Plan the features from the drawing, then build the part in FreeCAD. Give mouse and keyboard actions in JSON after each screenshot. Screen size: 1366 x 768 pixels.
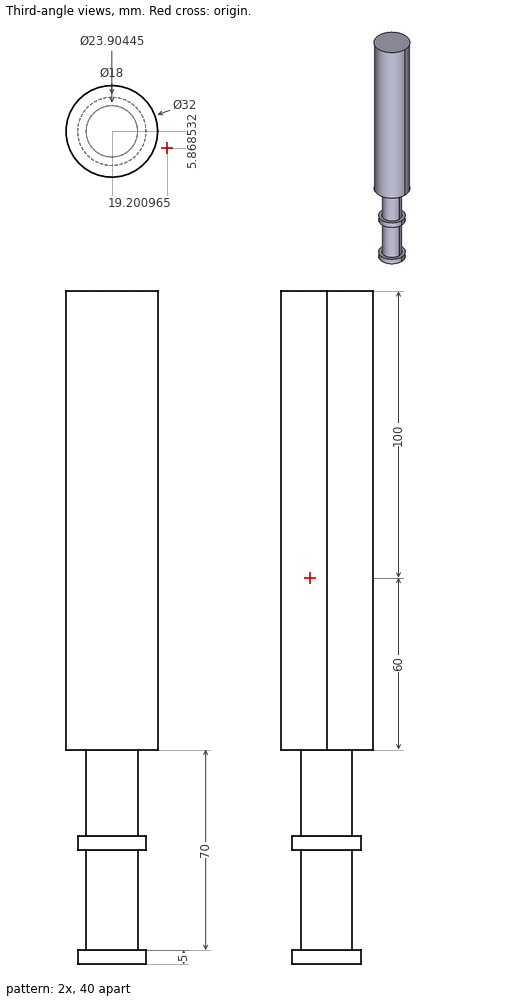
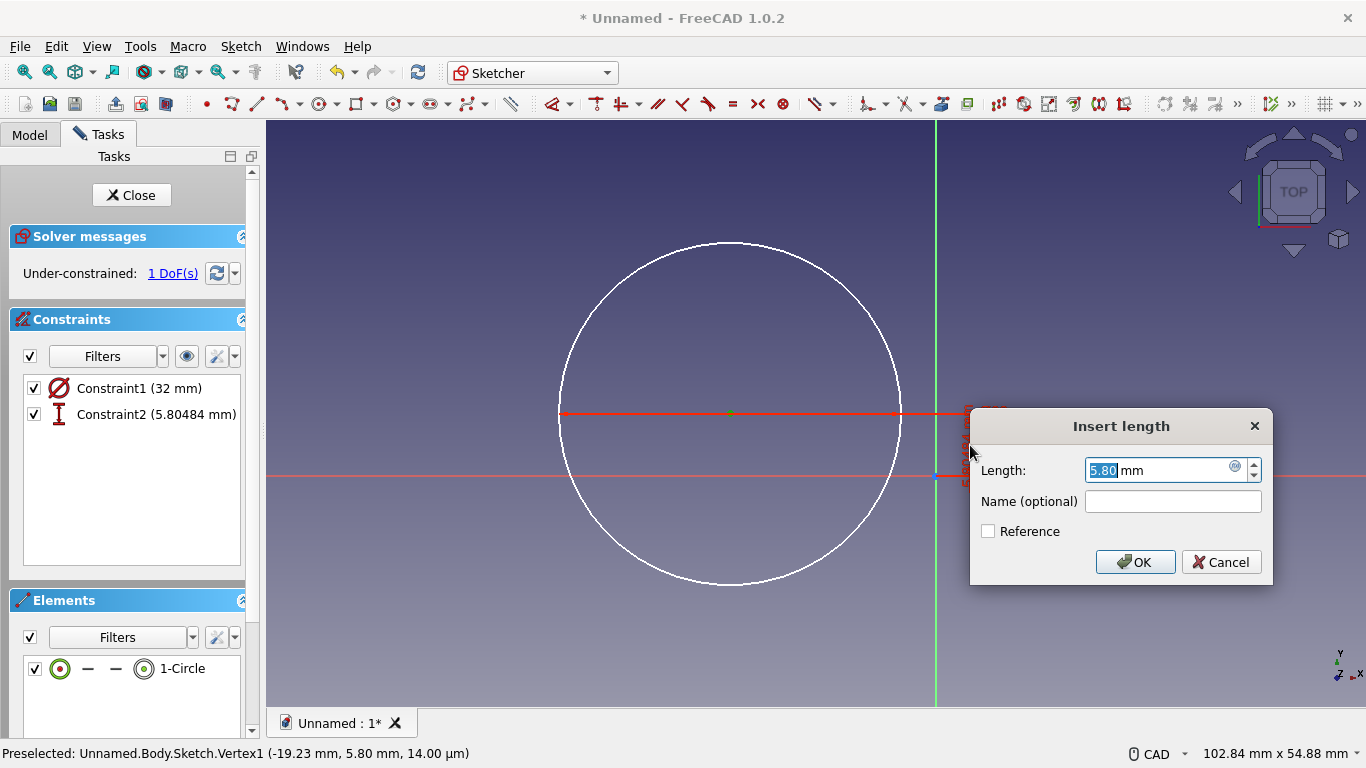
{"action": "type", "text": "5.868532"}
{"action": "key", "text": "Return"}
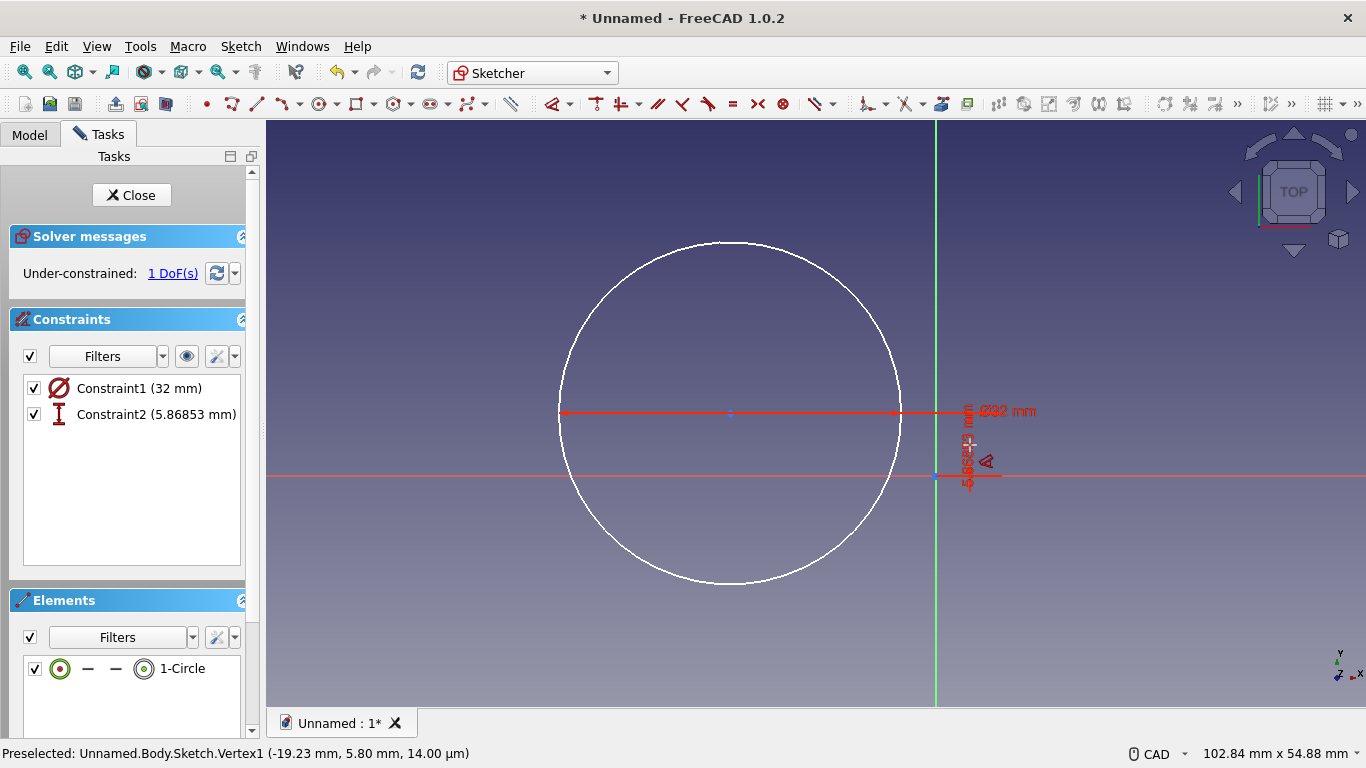
{"action": "left_click", "coordinate": [730, 413]}
{"action": "left_click", "coordinate": [833, 510]}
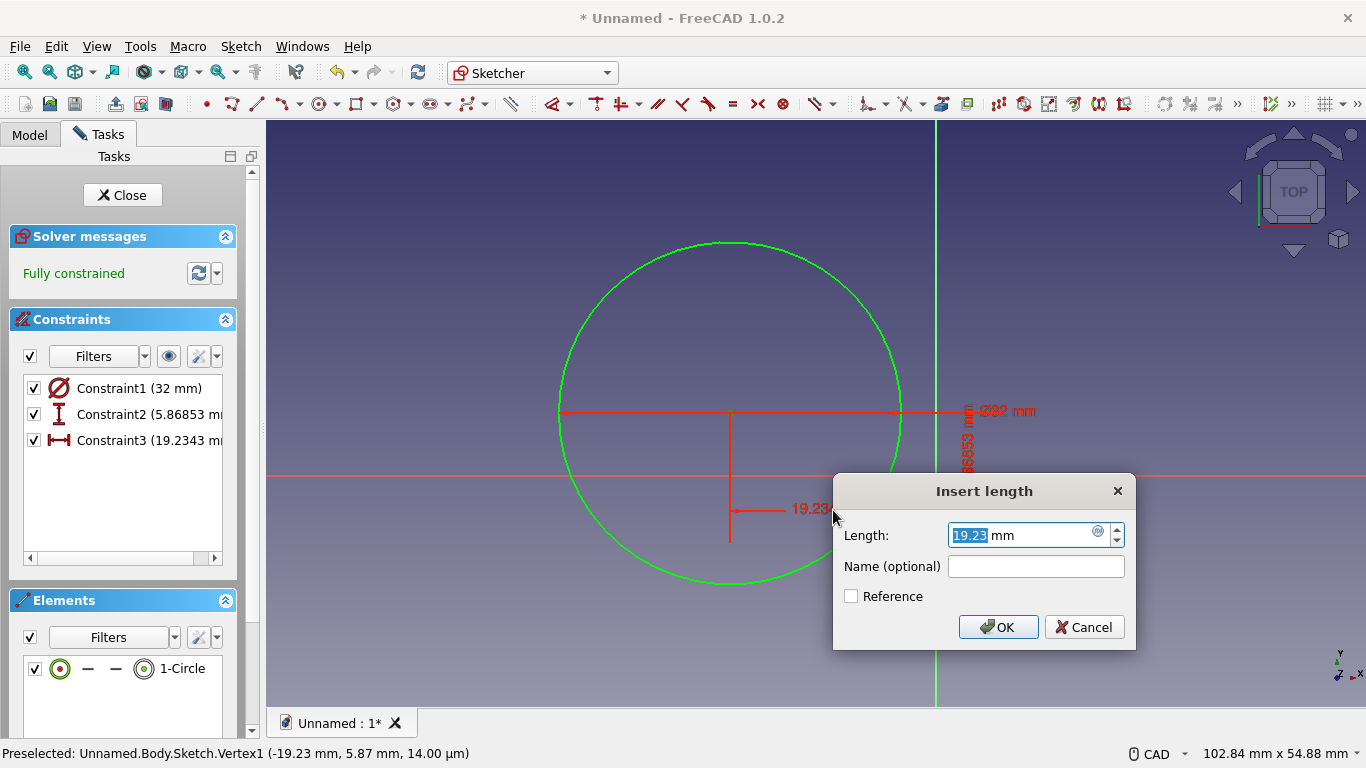
{"action": "type", "text": "19.200965"}
{"action": "key", "text": "Return"}
{"action": "key", "text": "Escape"}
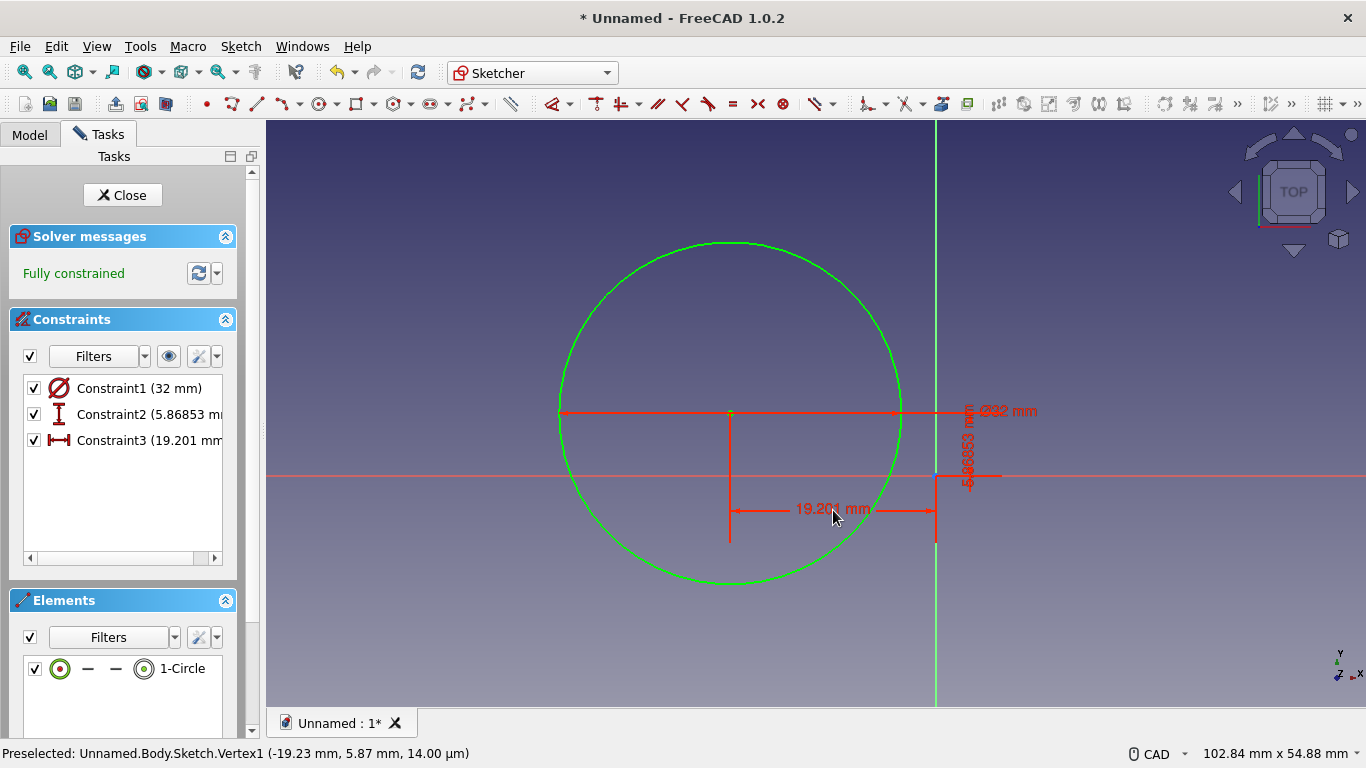
{"action": "left_click", "coordinate": [123, 195]}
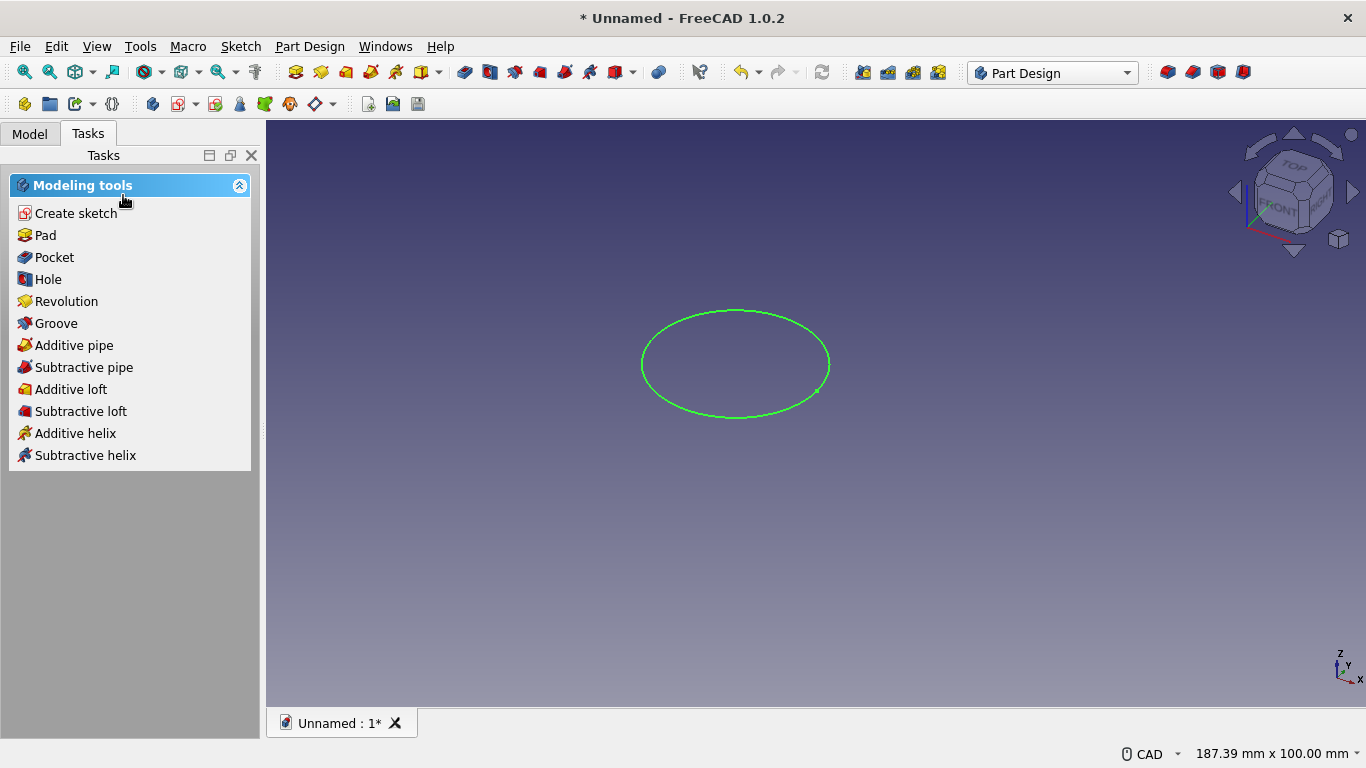
{"action": "left_click", "coordinate": [296, 72]}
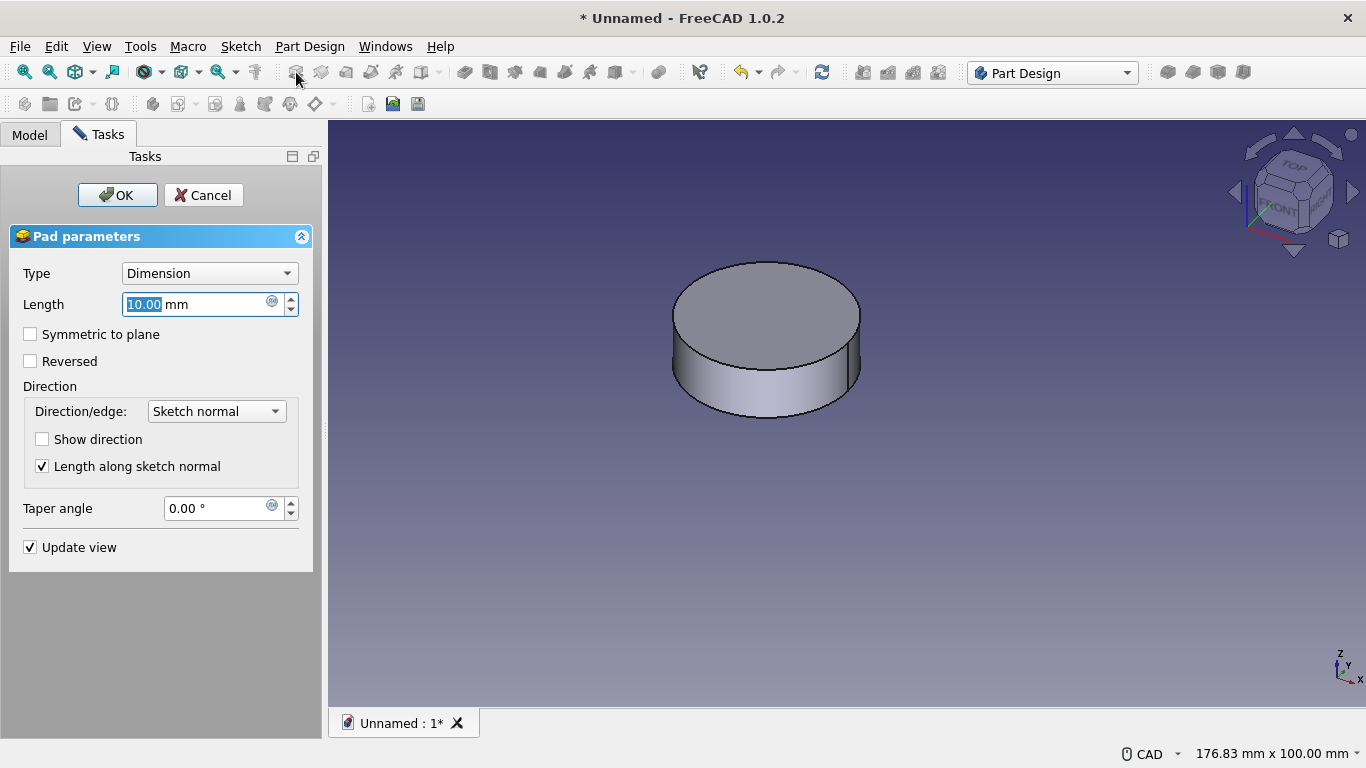
{"action": "type", "text": "60"}
{"action": "key", "text": "Tab"}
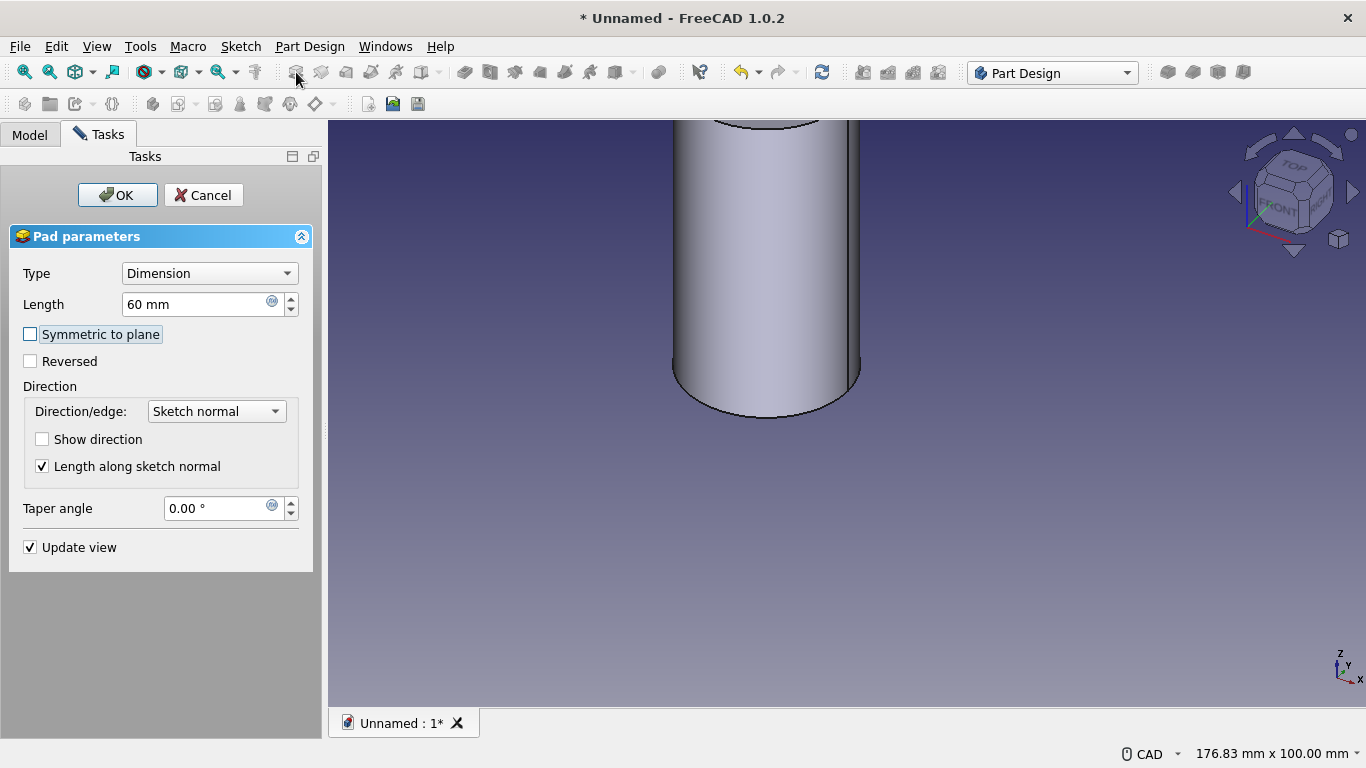
{"action": "left_click", "coordinate": [31, 361]}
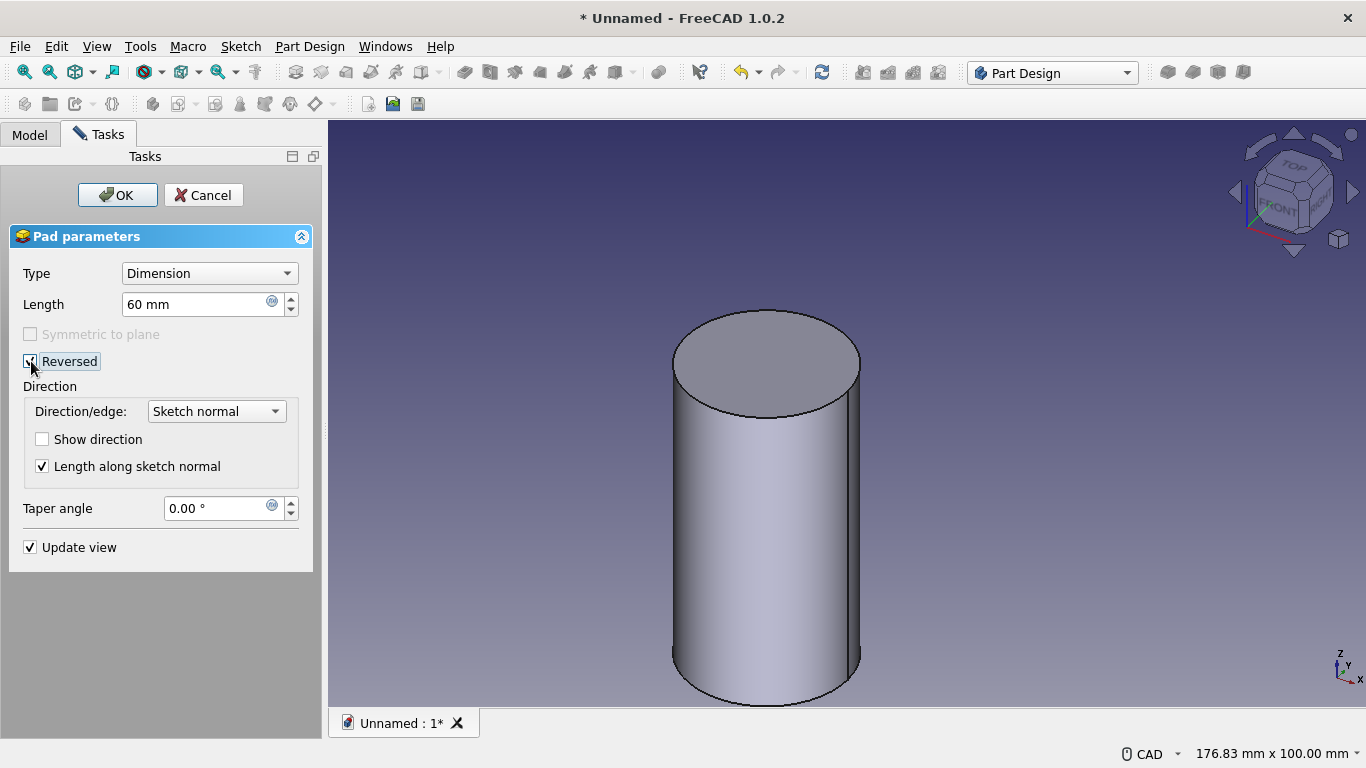
{"action": "left_click", "coordinate": [118, 195]}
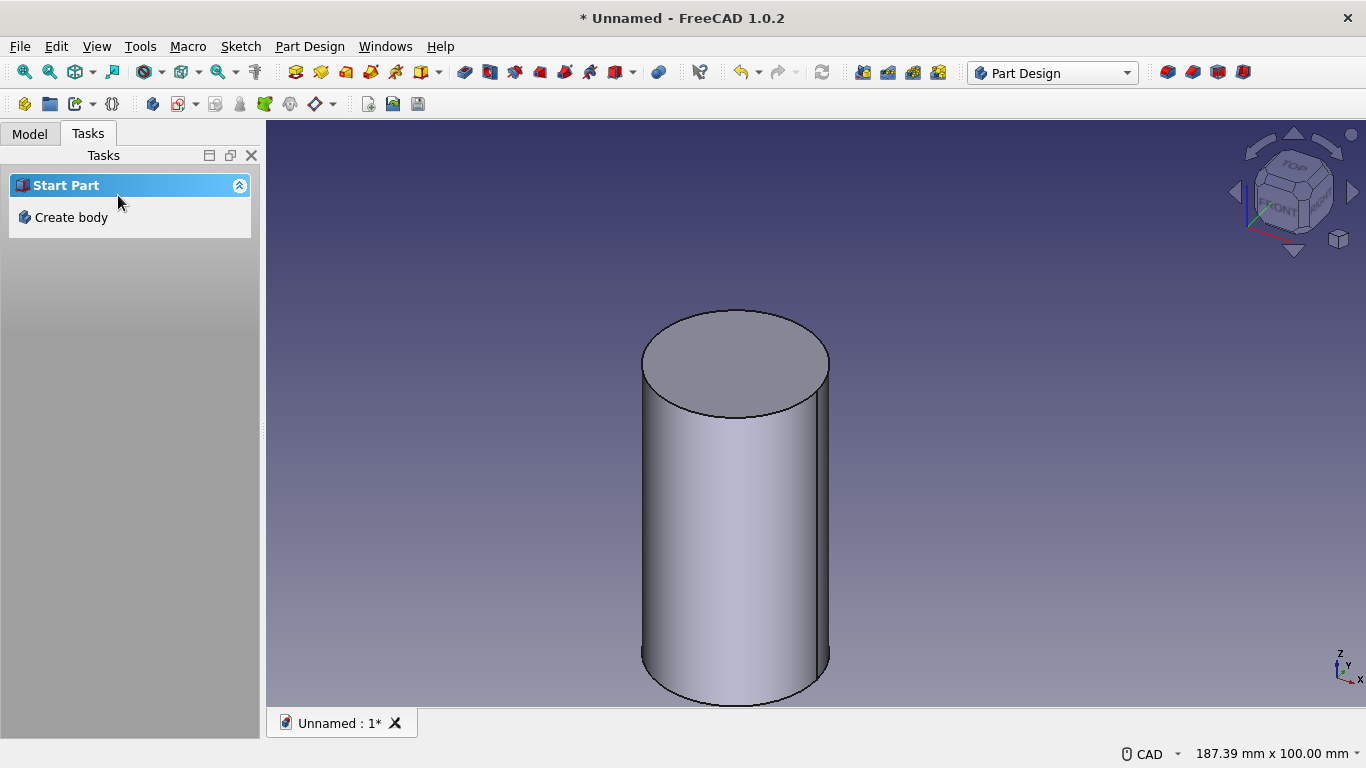
{"action": "key", "text": "v f"}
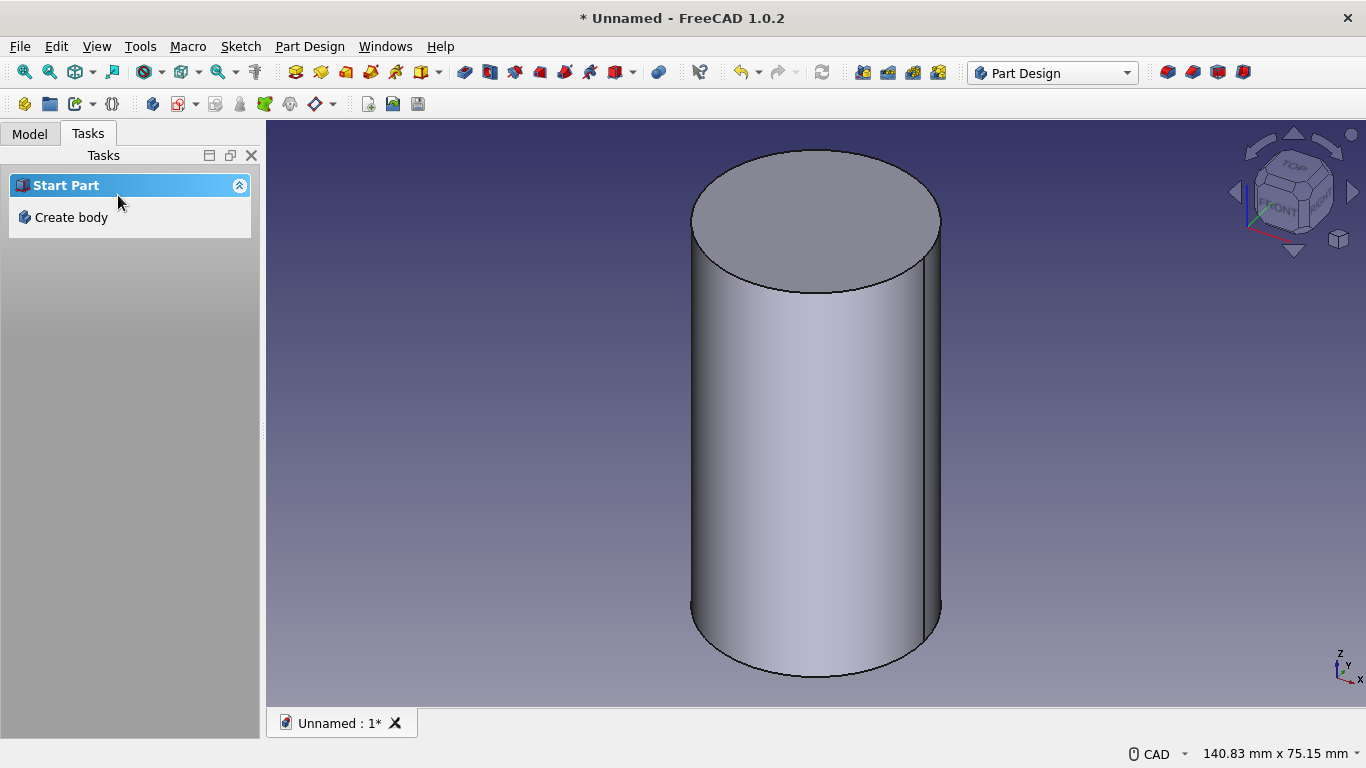
{"action": "key", "text": "5"}